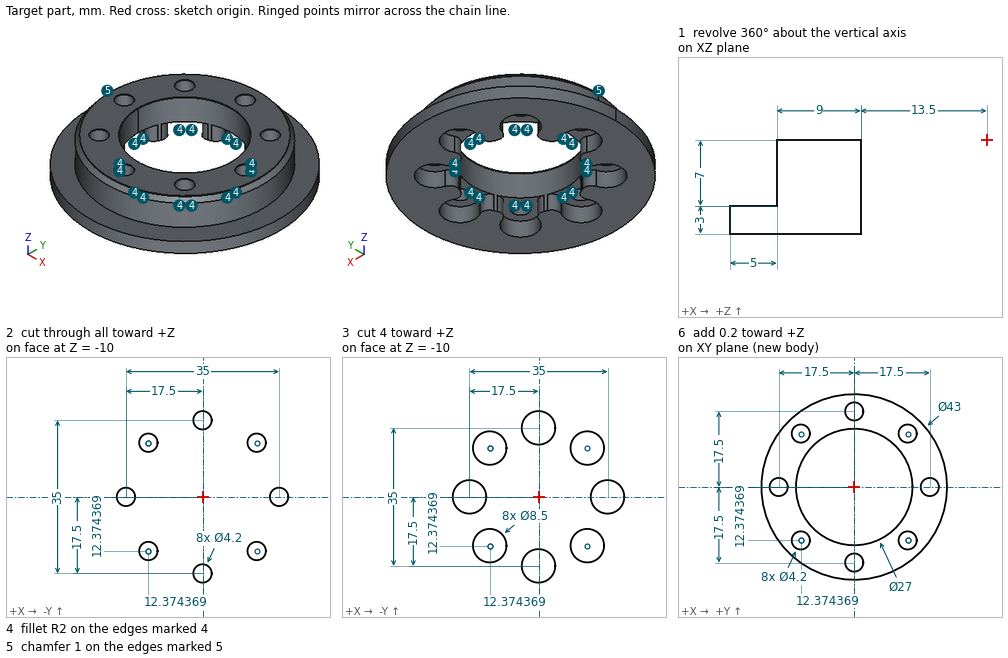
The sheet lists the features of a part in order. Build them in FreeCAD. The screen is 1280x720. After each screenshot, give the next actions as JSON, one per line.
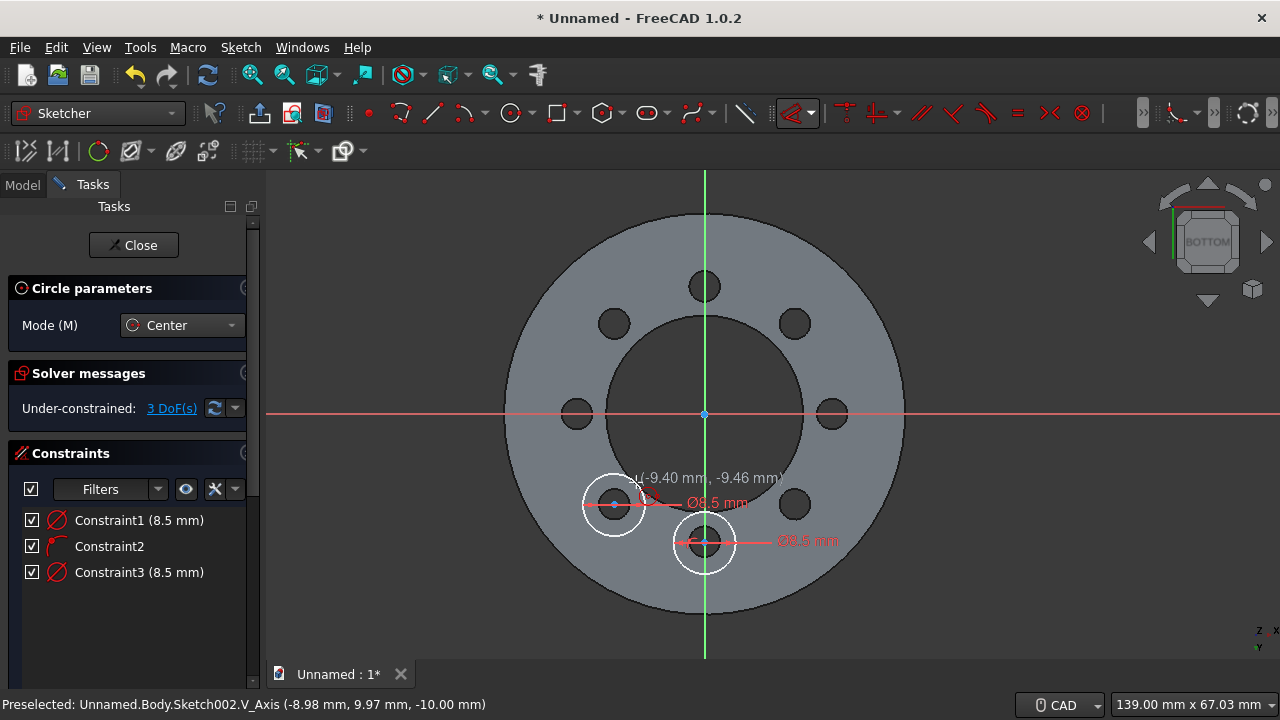
{"action": "left_click", "coordinate": [577, 414]}
{"action": "mouse_move", "coordinate": [599, 392]}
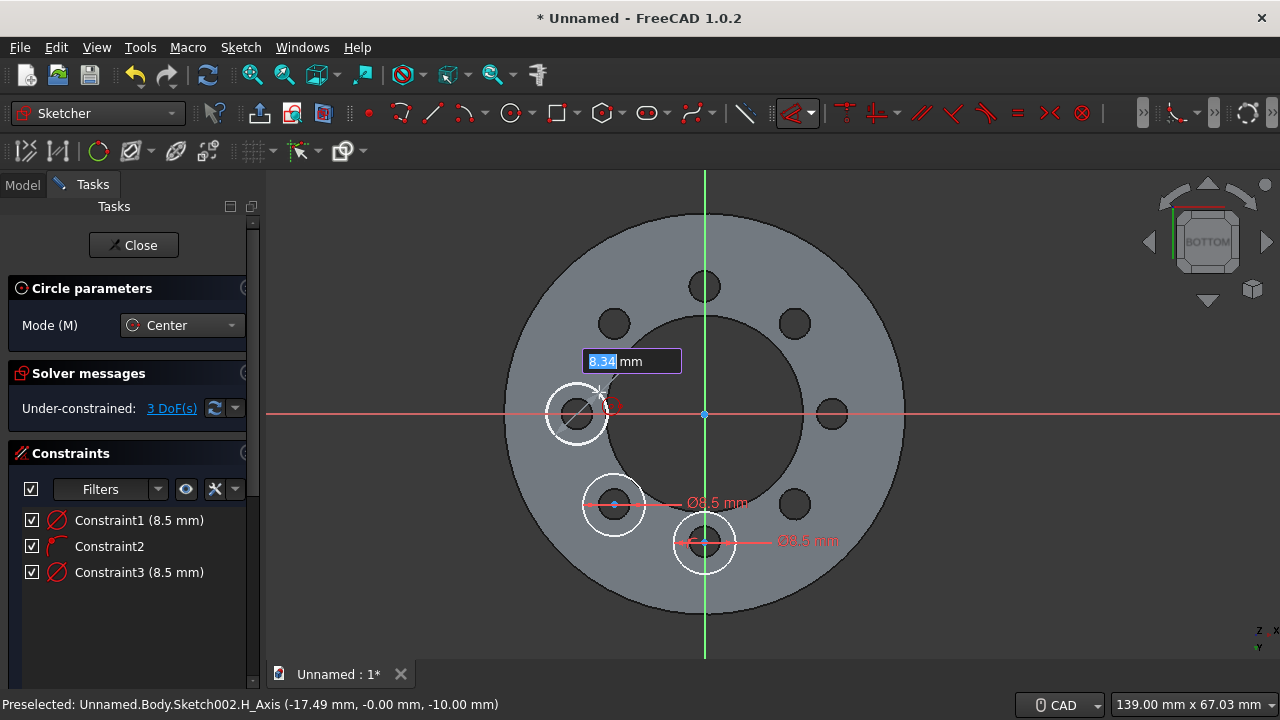
{"action": "type", "text": "8.5"}
{"action": "key", "text": "Return"}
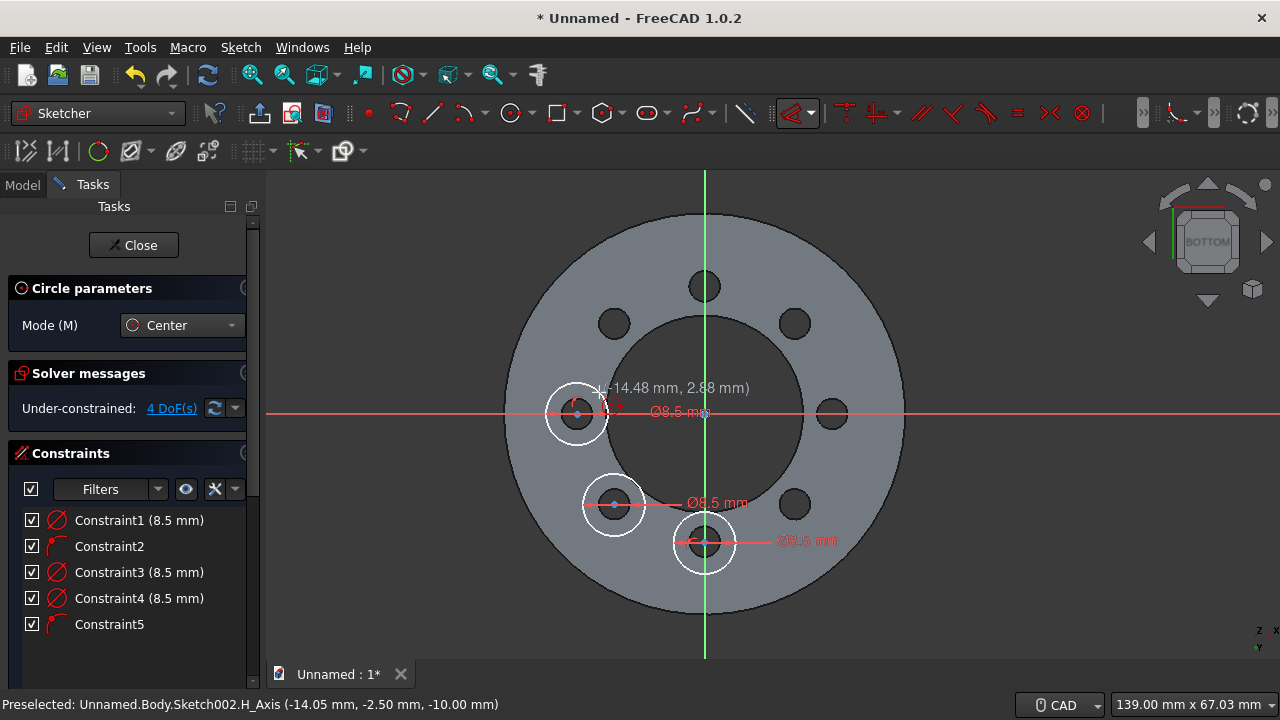
{"action": "left_click", "coordinate": [614, 324]}
{"action": "mouse_move", "coordinate": [636, 302]}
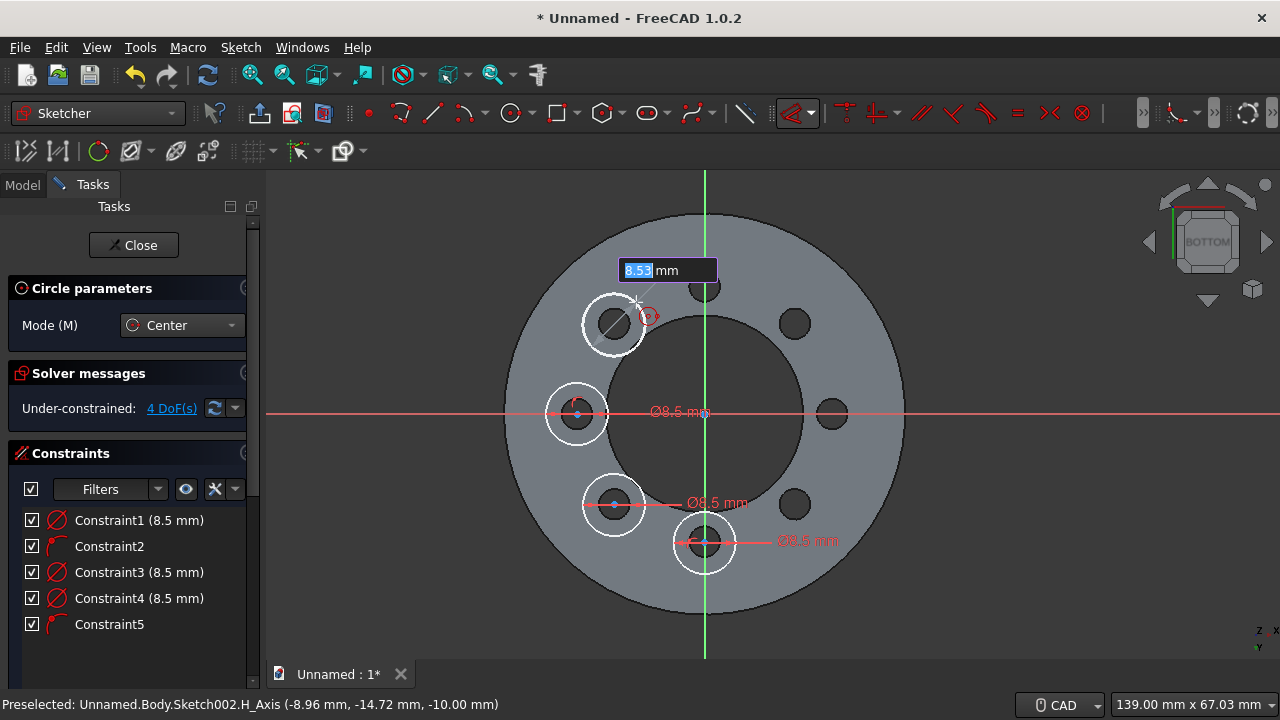
{"action": "type", "text": "8.5"}
{"action": "key", "text": "Return"}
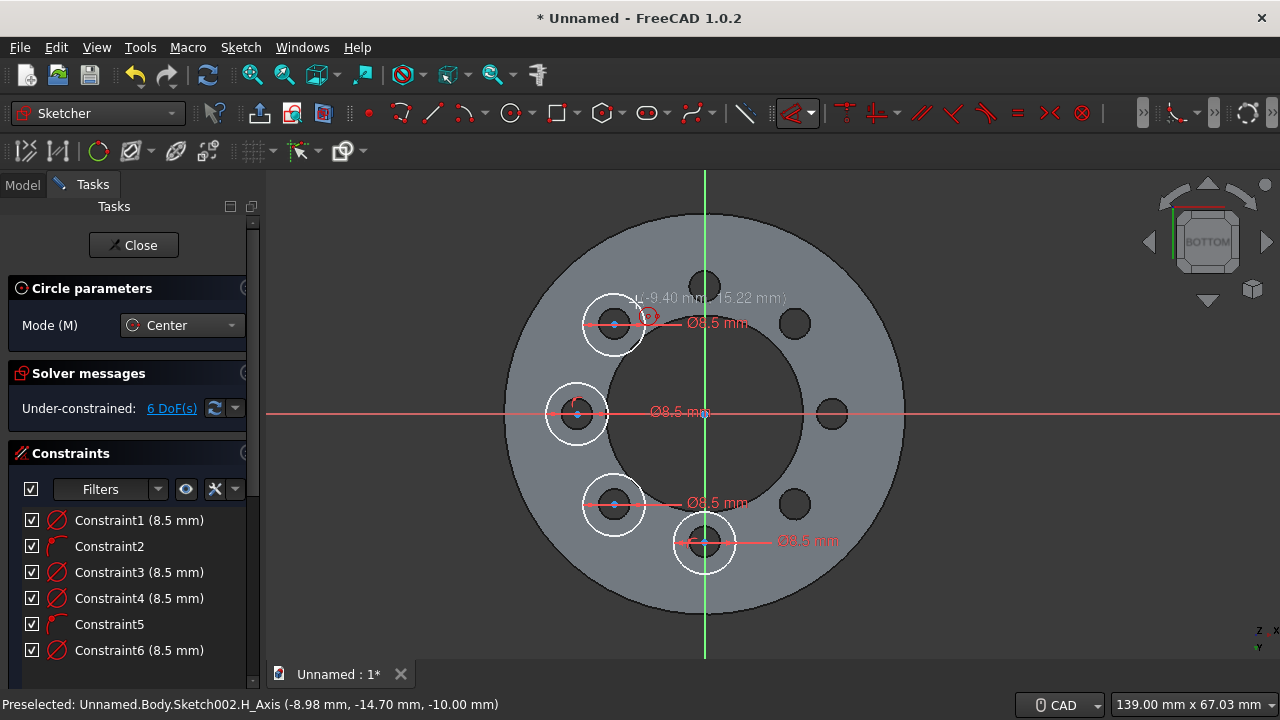
{"action": "left_click", "coordinate": [705, 286]}
{"action": "mouse_move", "coordinate": [727, 264]}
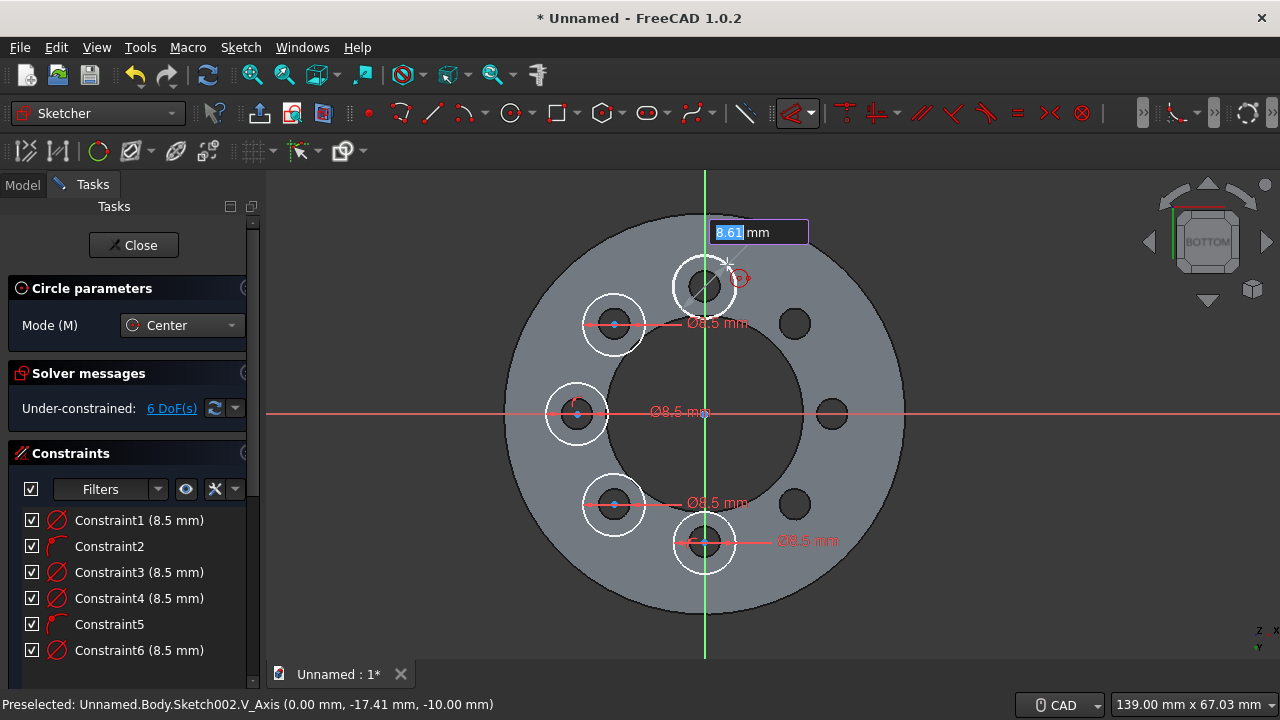
{"action": "type", "text": "8.5"}
{"action": "key", "text": "Return"}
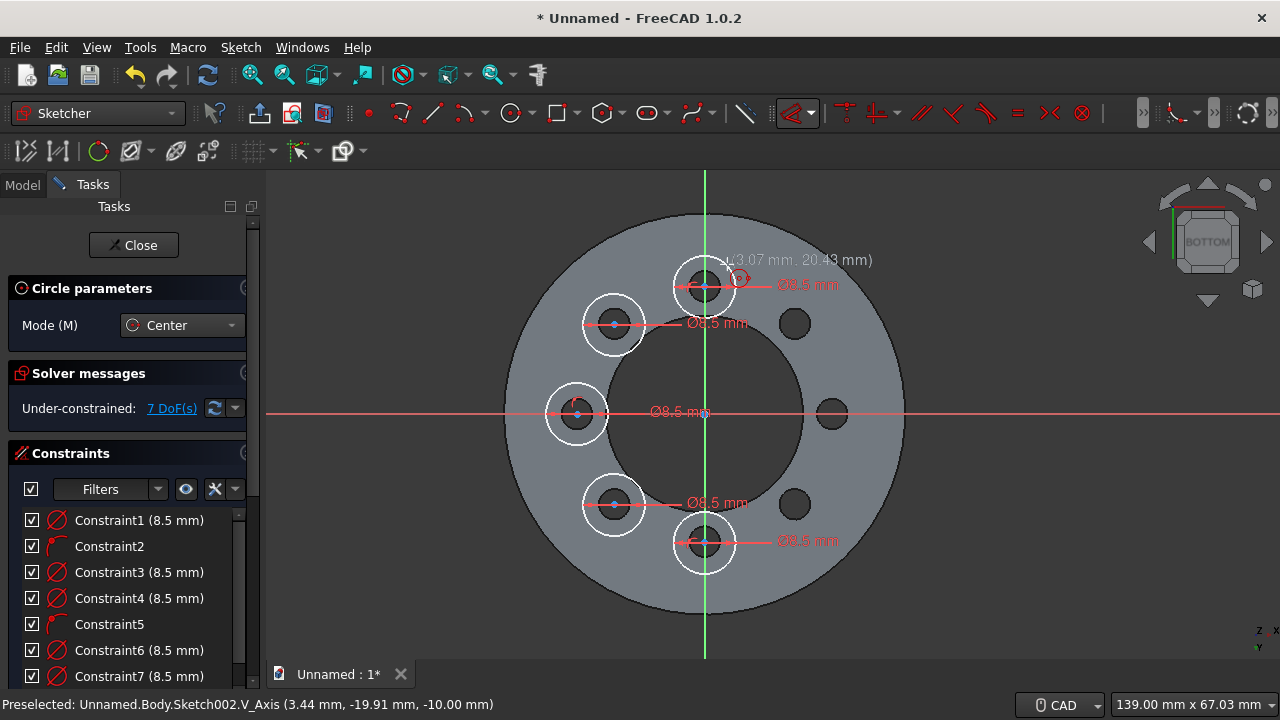
{"action": "left_click", "coordinate": [795, 324]}
{"action": "mouse_move", "coordinate": [817, 302]}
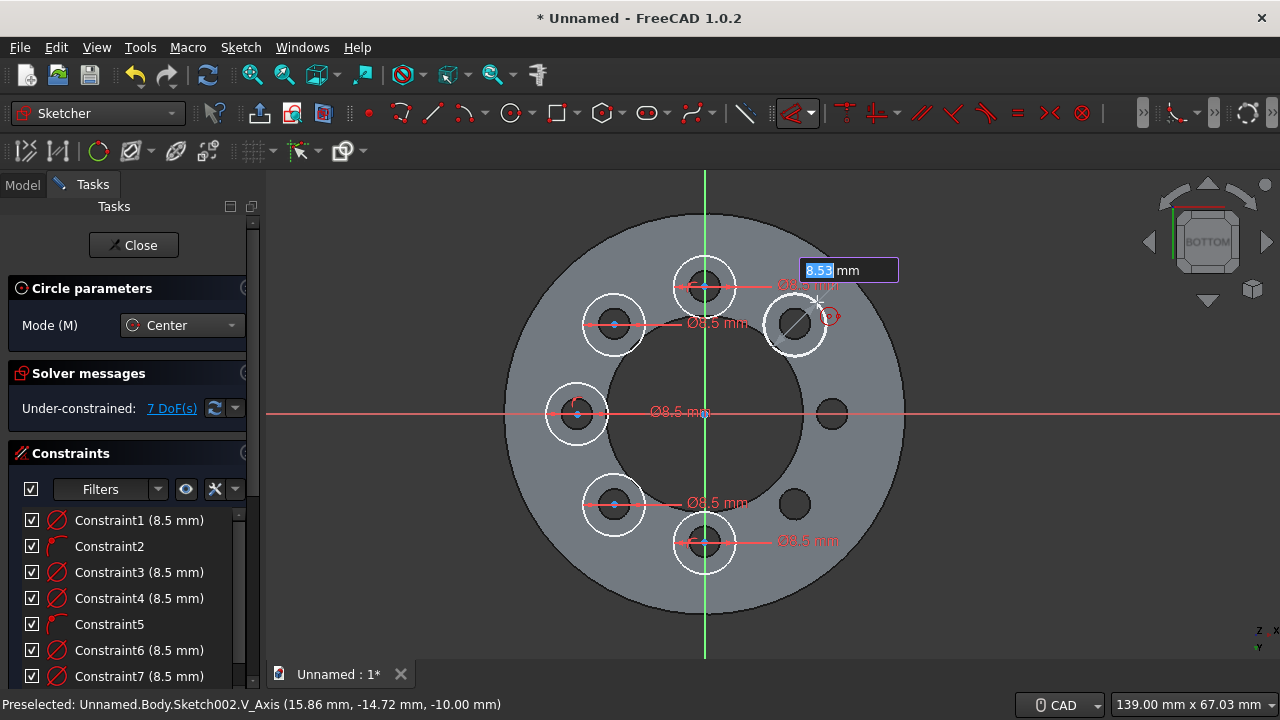
{"action": "type", "text": "8.5"}
{"action": "key", "text": "Return"}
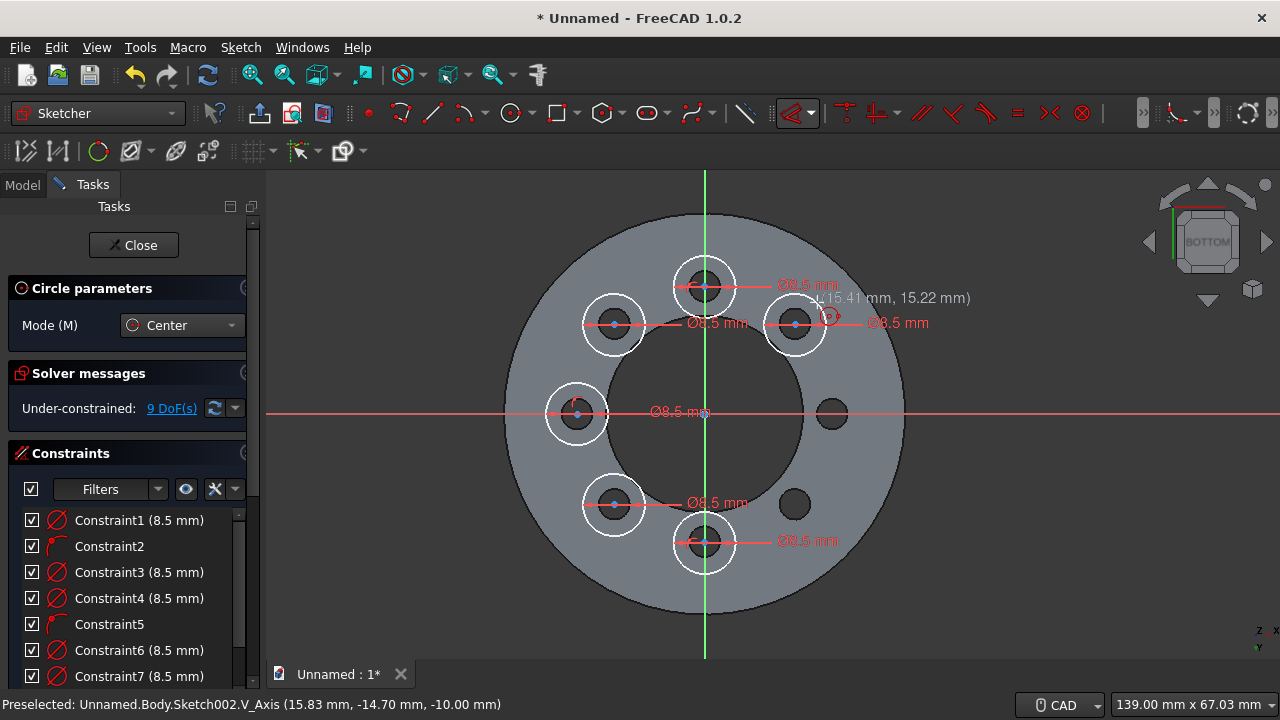
{"action": "left_click", "coordinate": [832, 414]}
{"action": "mouse_move", "coordinate": [854, 392]}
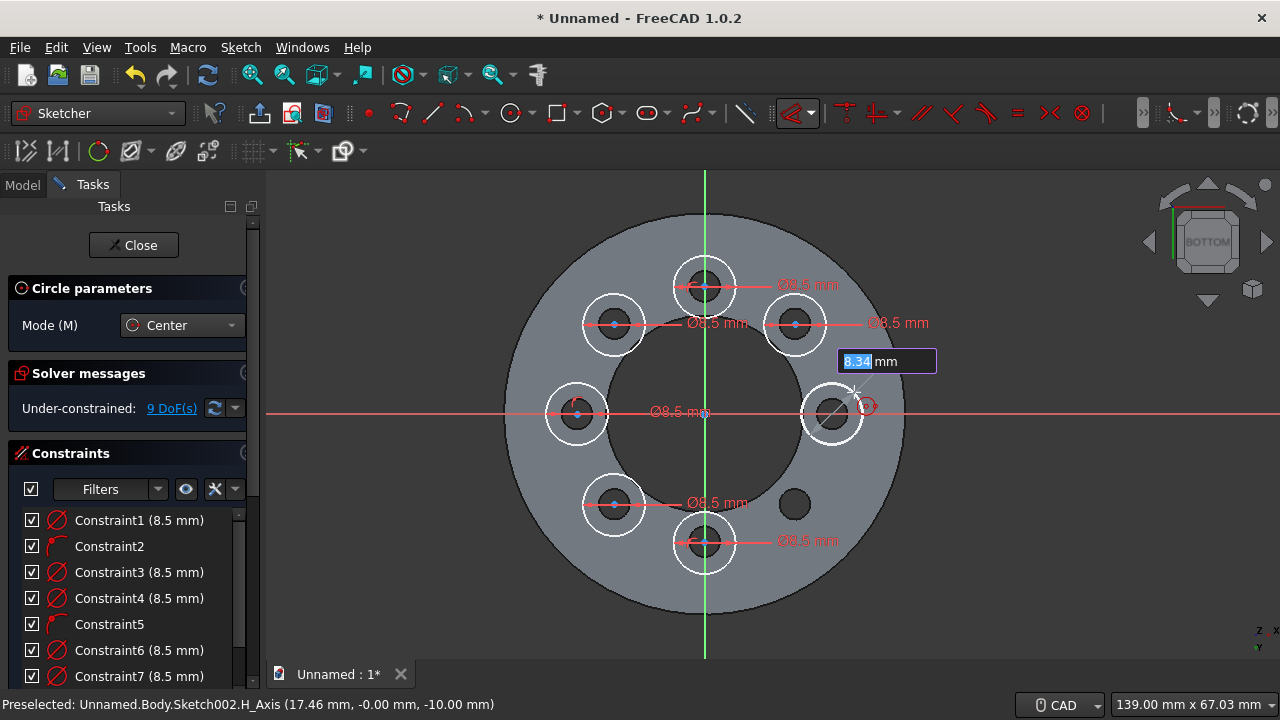
{"action": "type", "text": "8.5"}
{"action": "key", "text": "Return"}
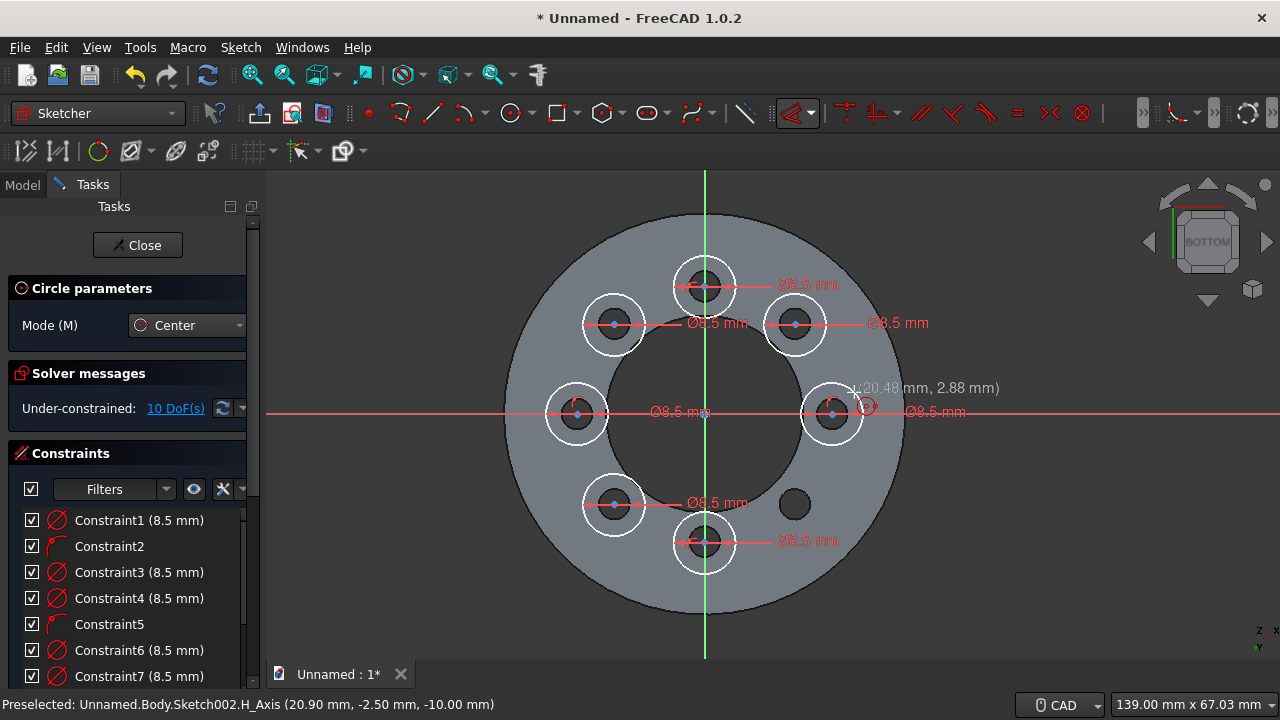
{"action": "left_click", "coordinate": [795, 504]}
{"action": "mouse_move", "coordinate": [817, 482]}